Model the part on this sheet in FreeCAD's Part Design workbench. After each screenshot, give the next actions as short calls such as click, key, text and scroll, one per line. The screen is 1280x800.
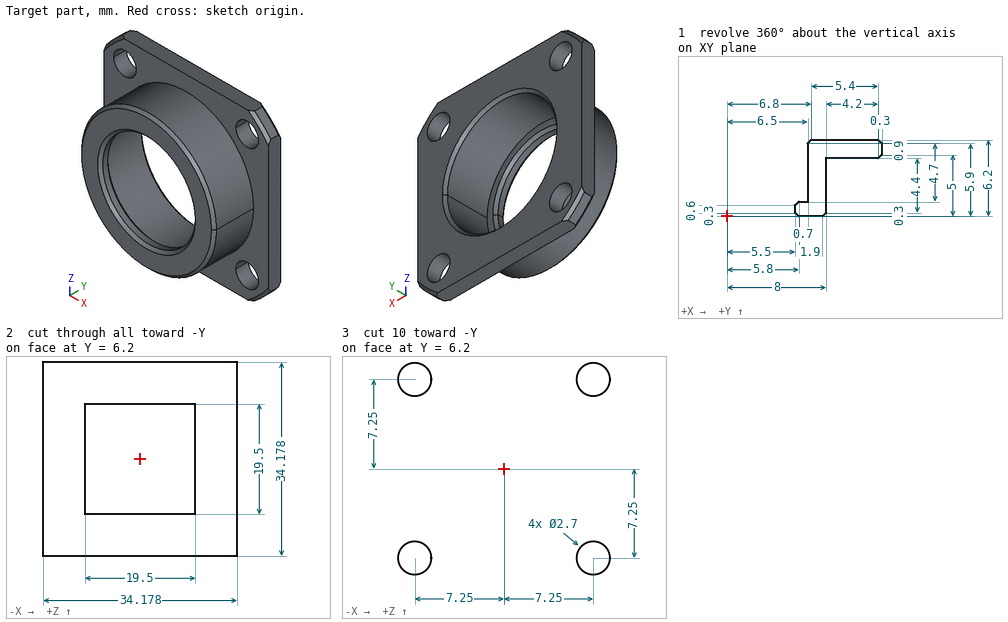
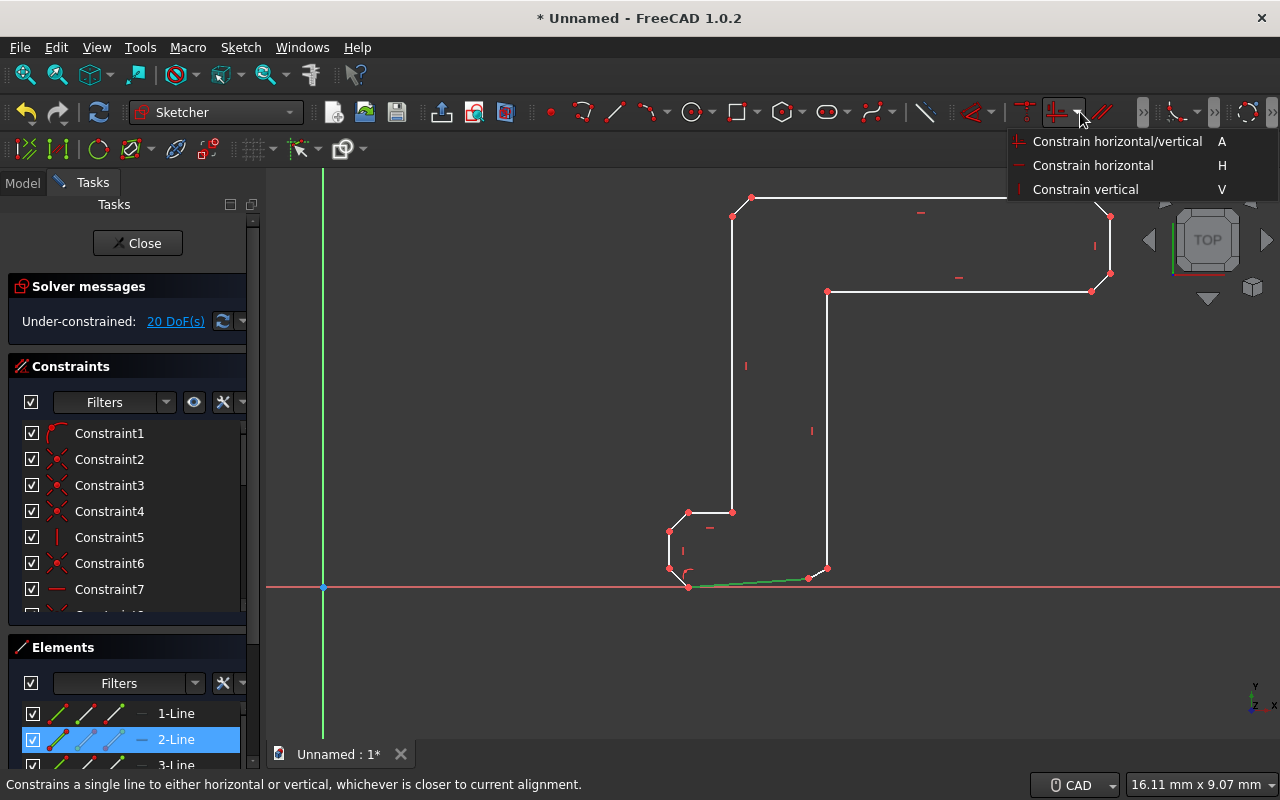
click(1143, 165)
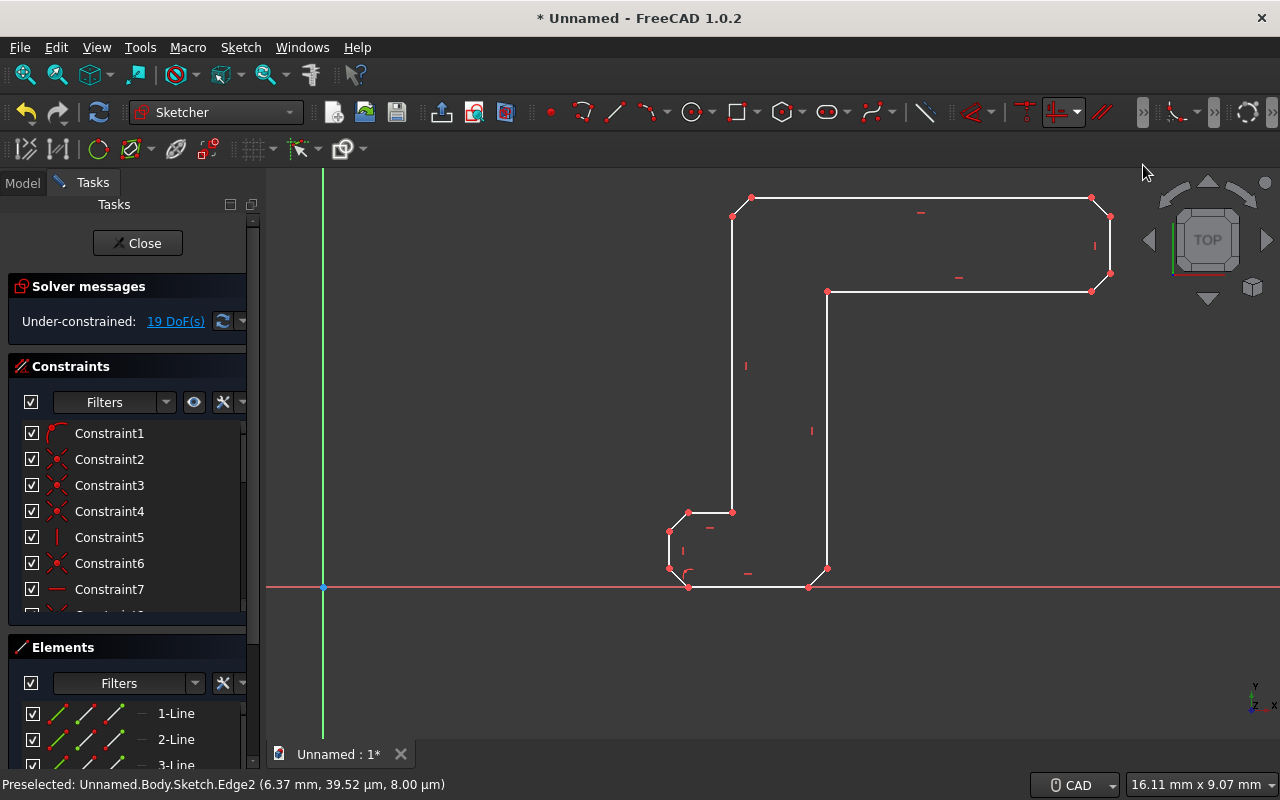
click(972, 112)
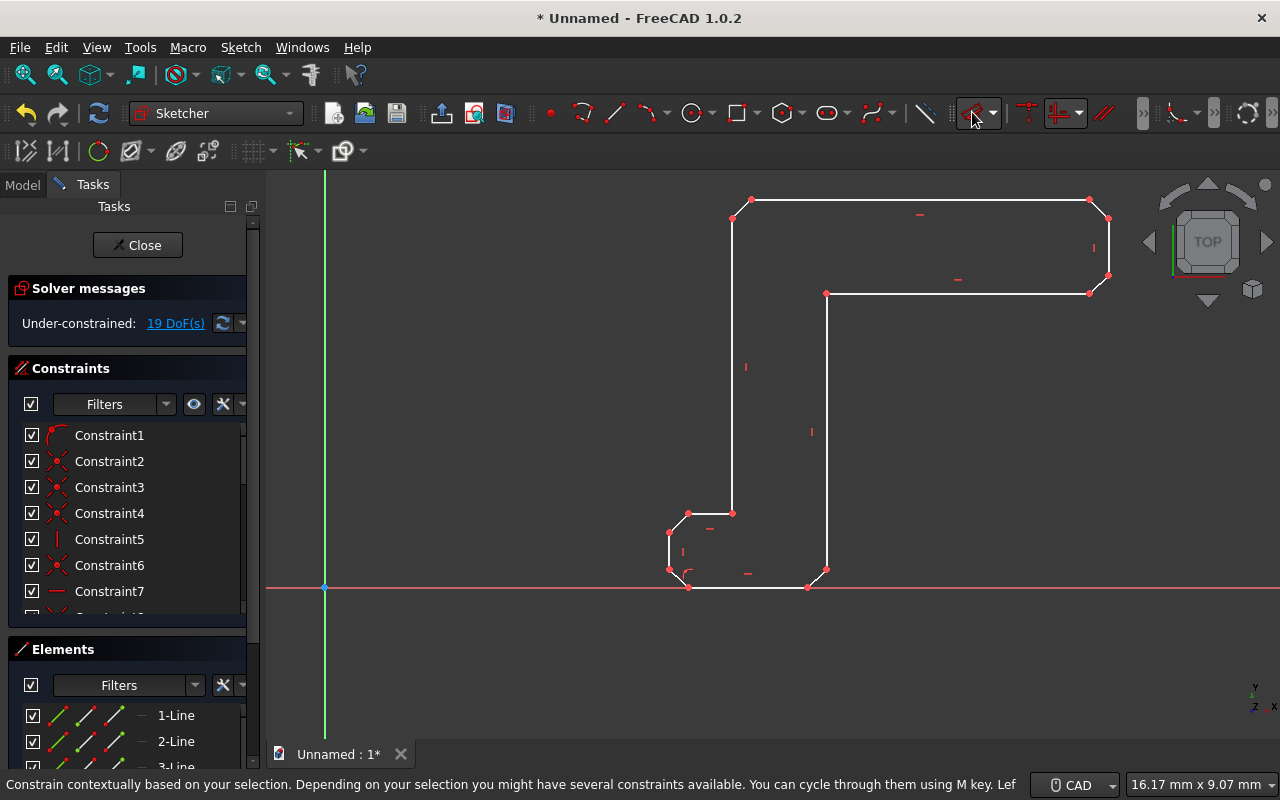
click(827, 570)
click(576, 622)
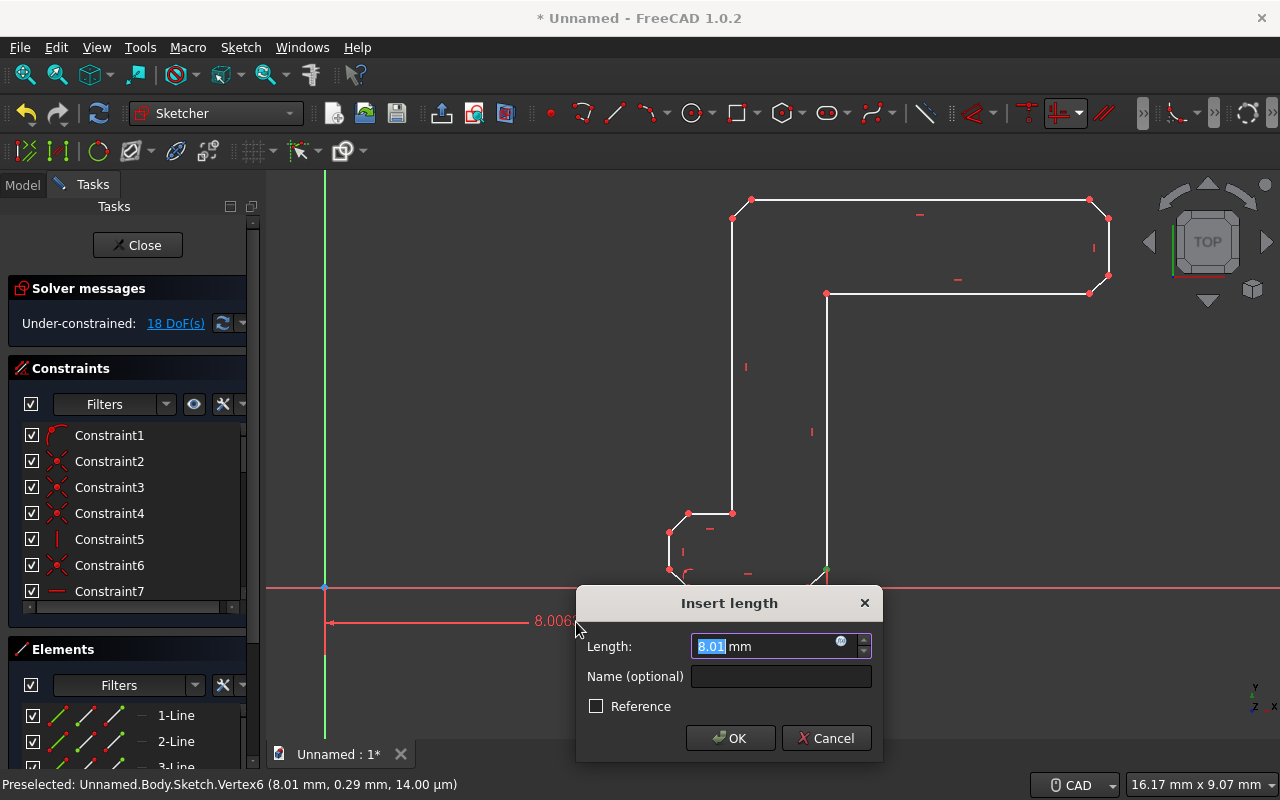
text(8)
key(Return)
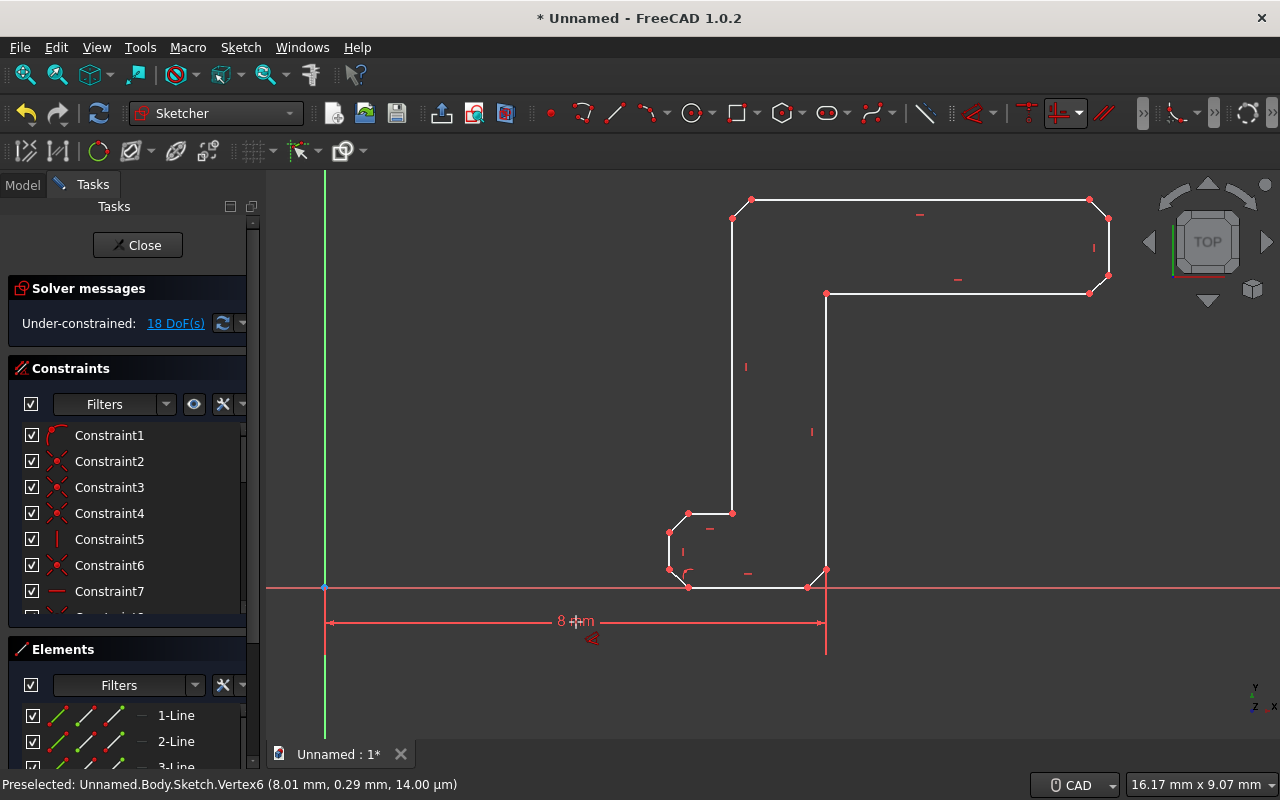
click(1109, 276)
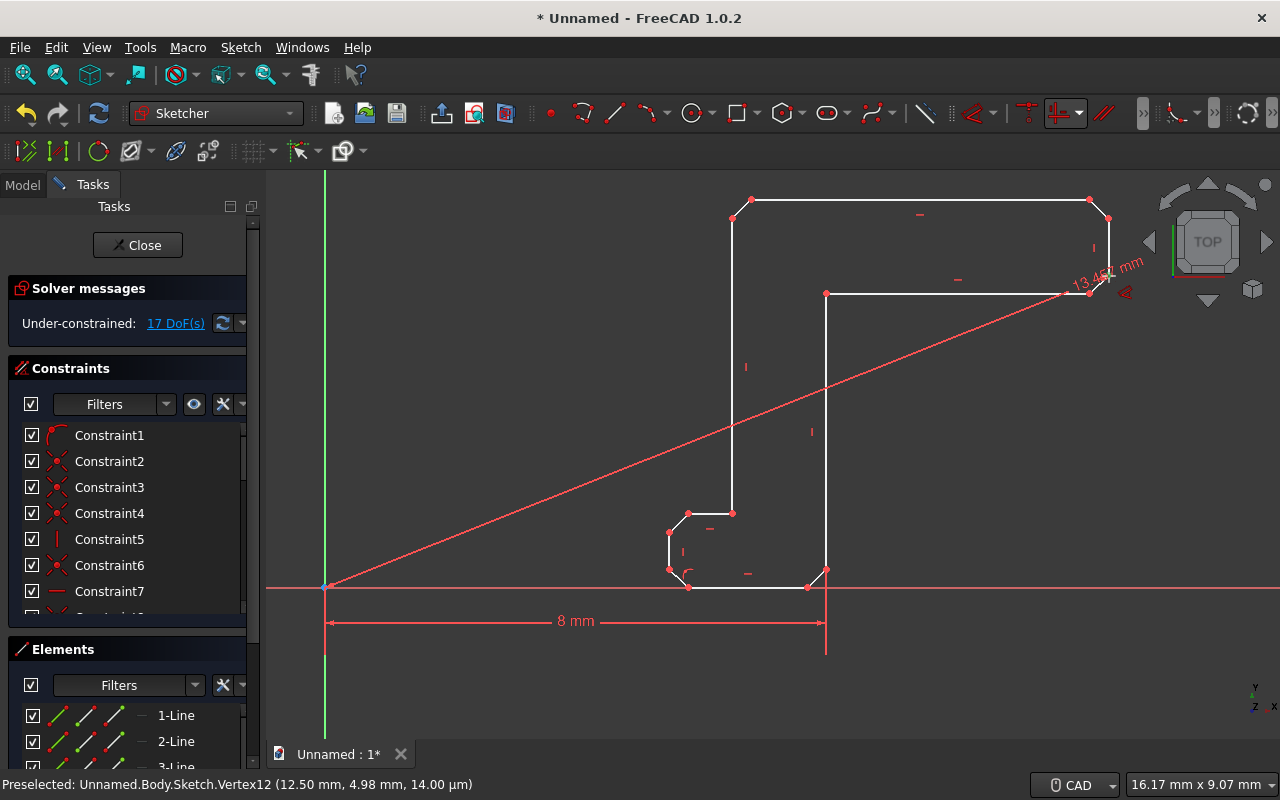
key(Escape)
key(Escape)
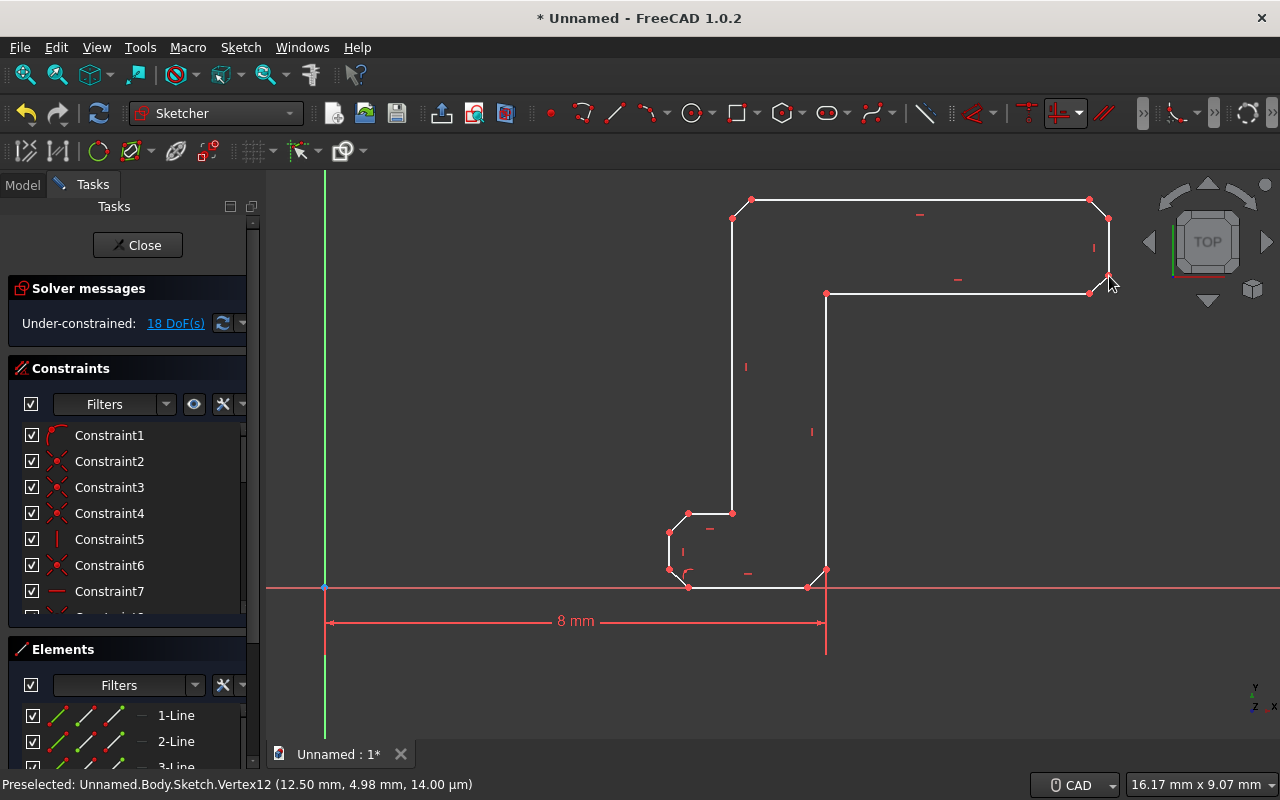
click(1109, 276)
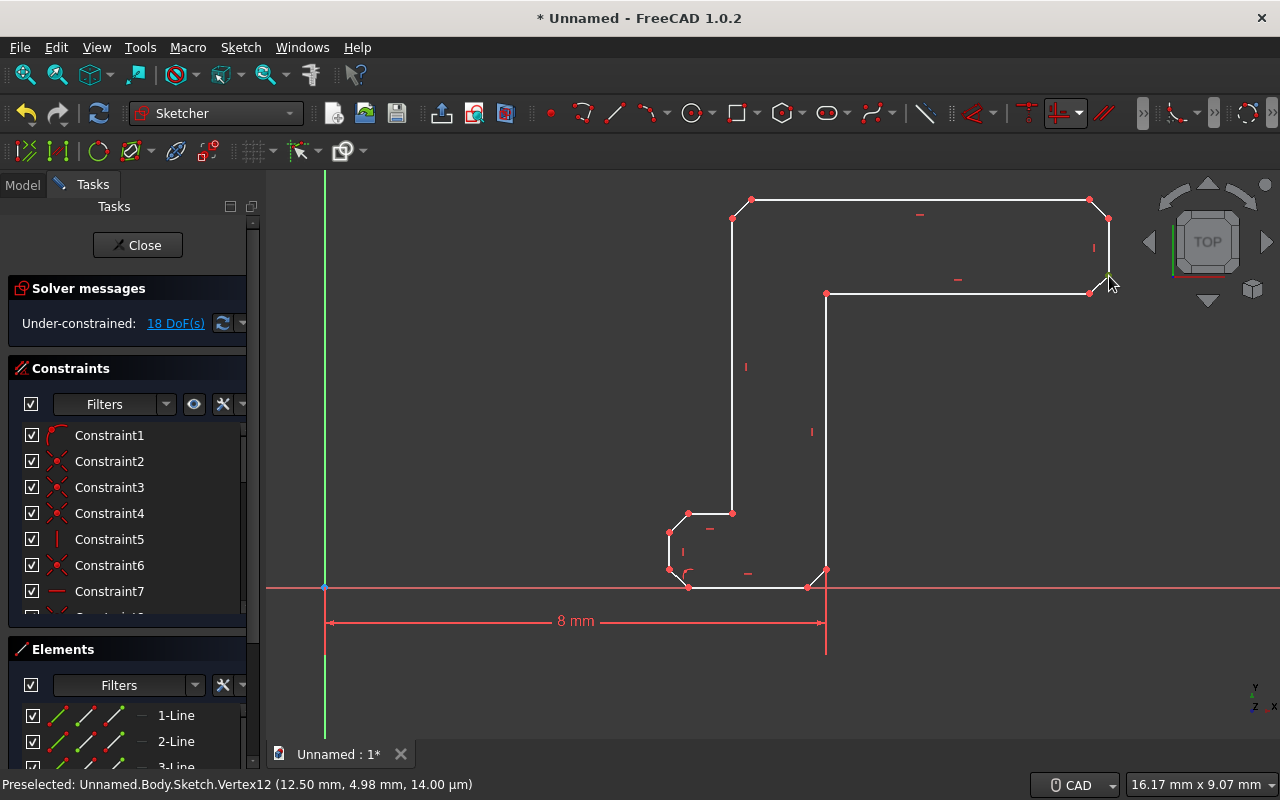
click(996, 114)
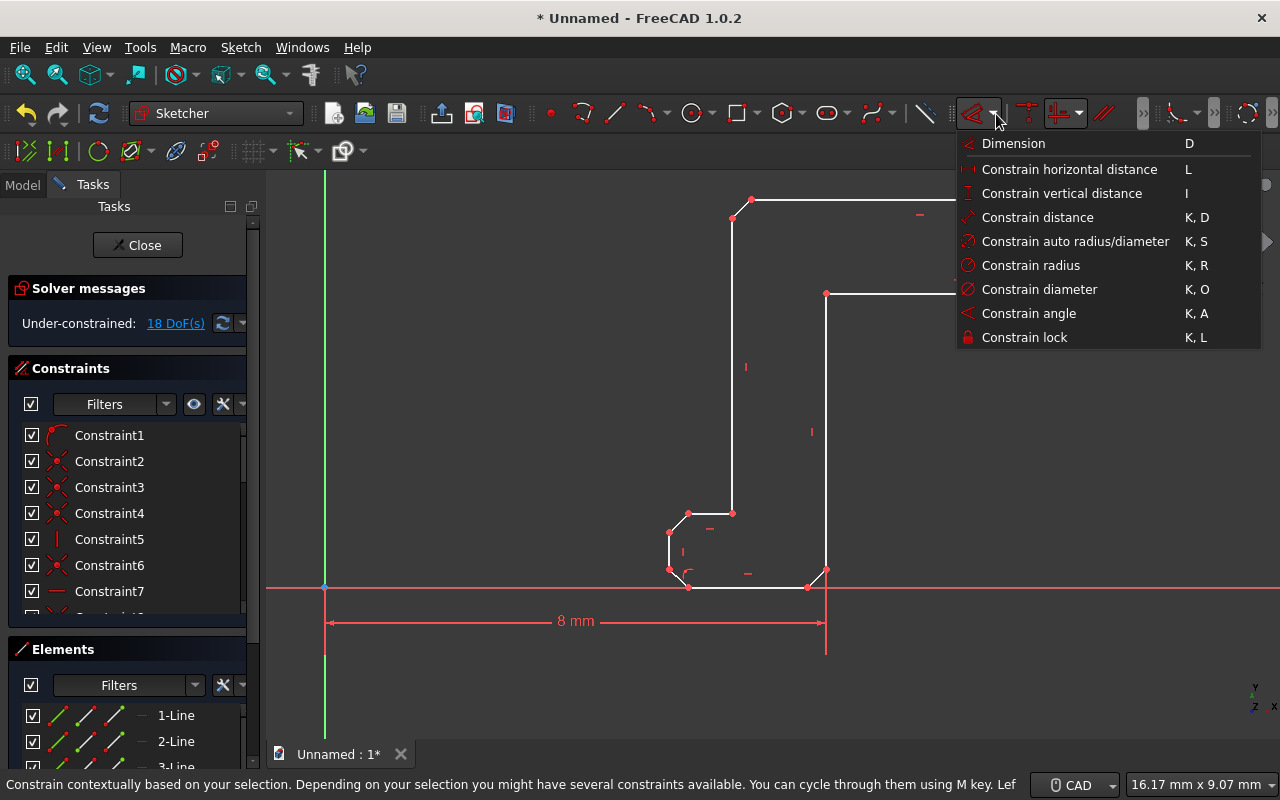
click(1109, 193)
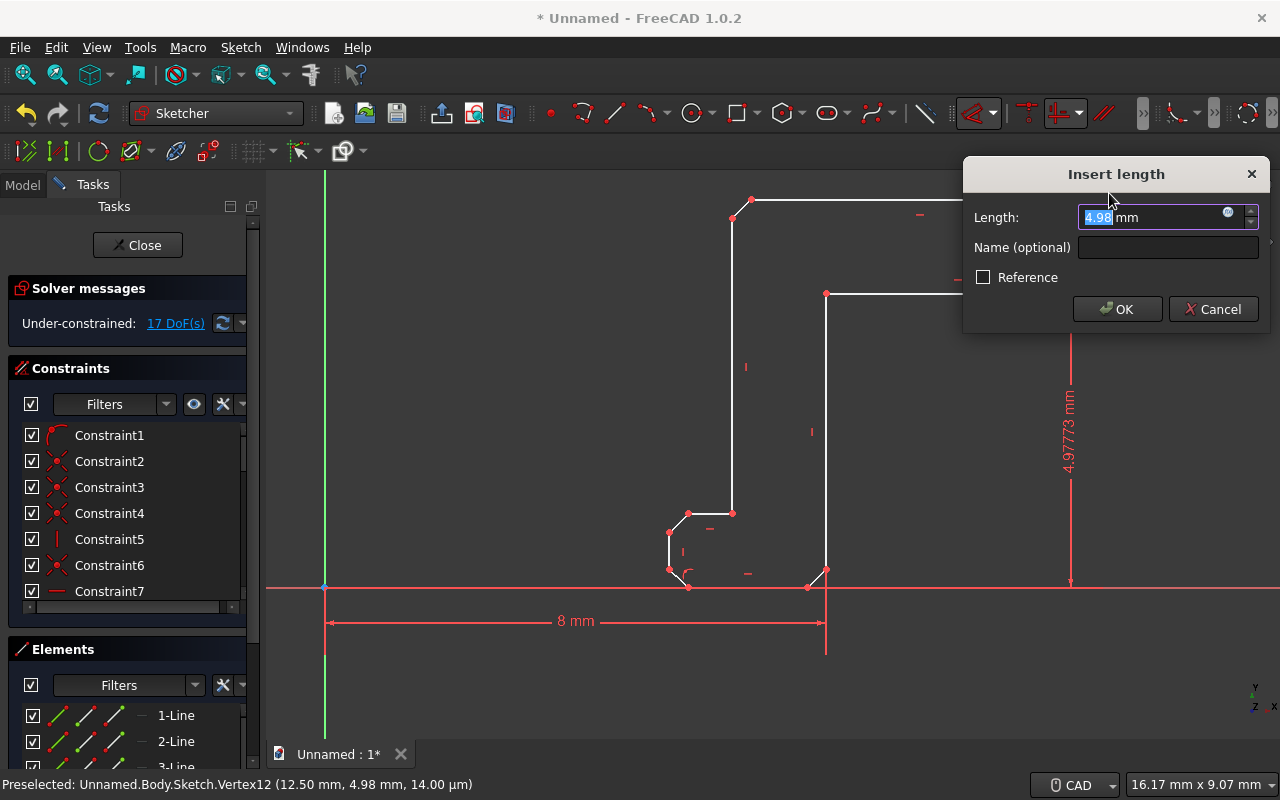
text(5)
key(Return)